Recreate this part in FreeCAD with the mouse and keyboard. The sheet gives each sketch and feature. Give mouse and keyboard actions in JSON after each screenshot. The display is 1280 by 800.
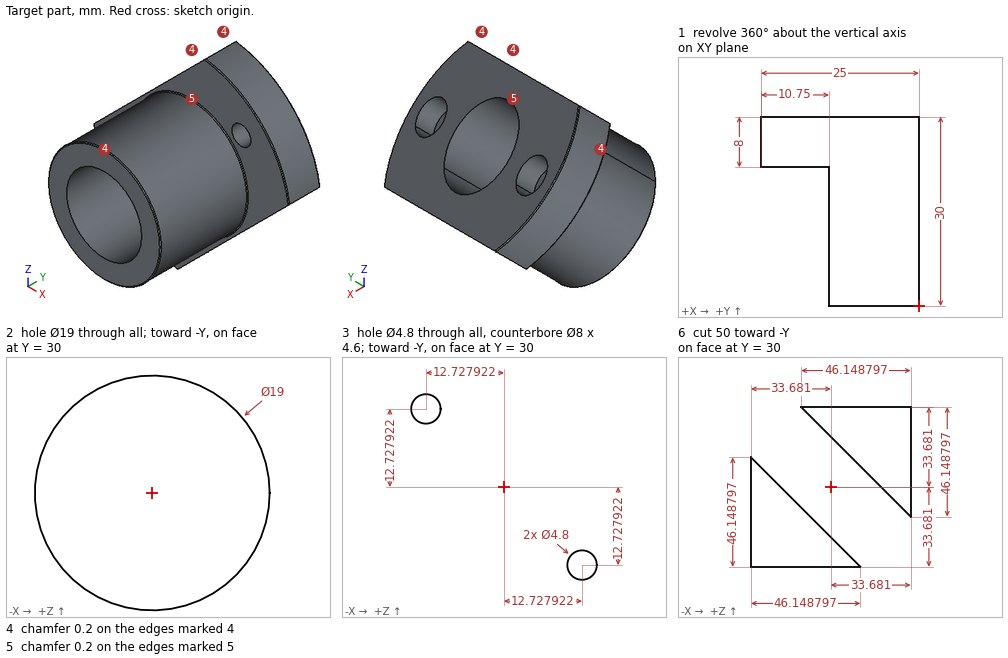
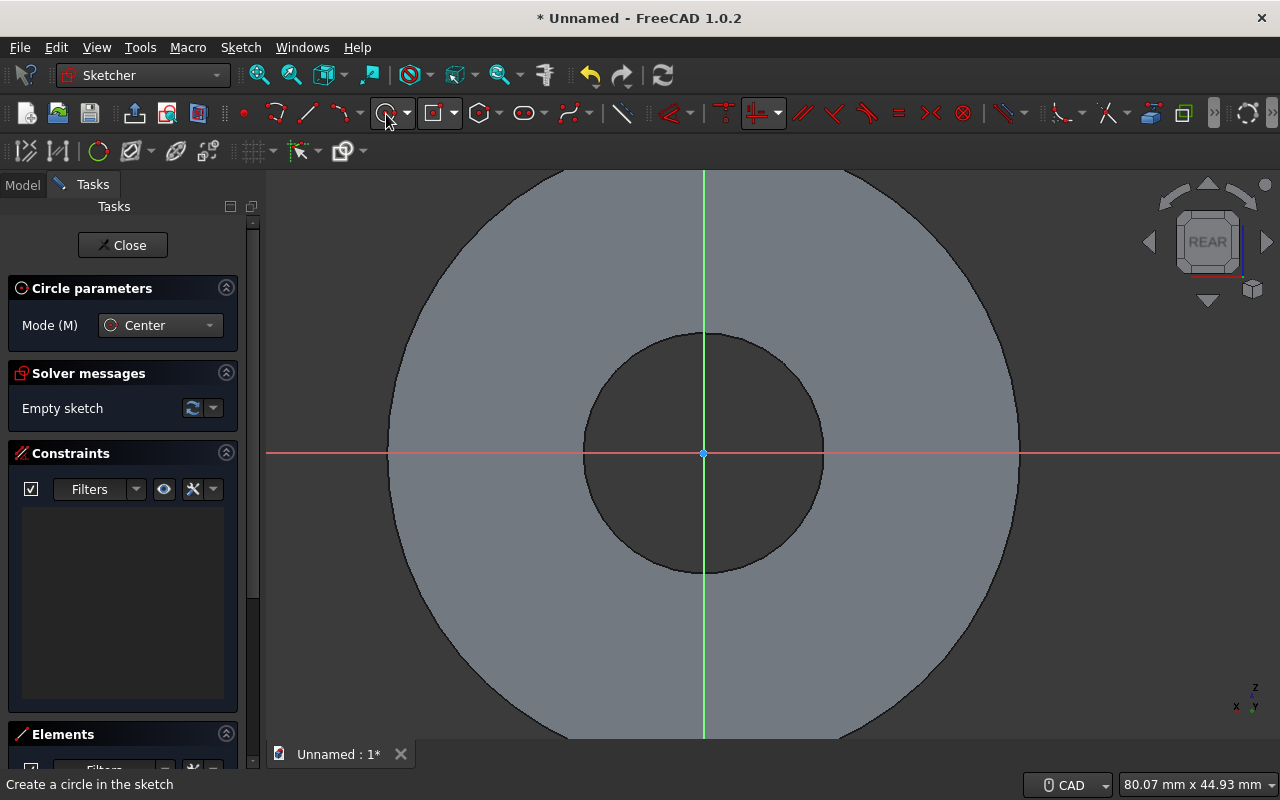
{"action": "left_click", "coordinate": [865, 614]}
{"action": "mouse_move", "coordinate": [886, 593]}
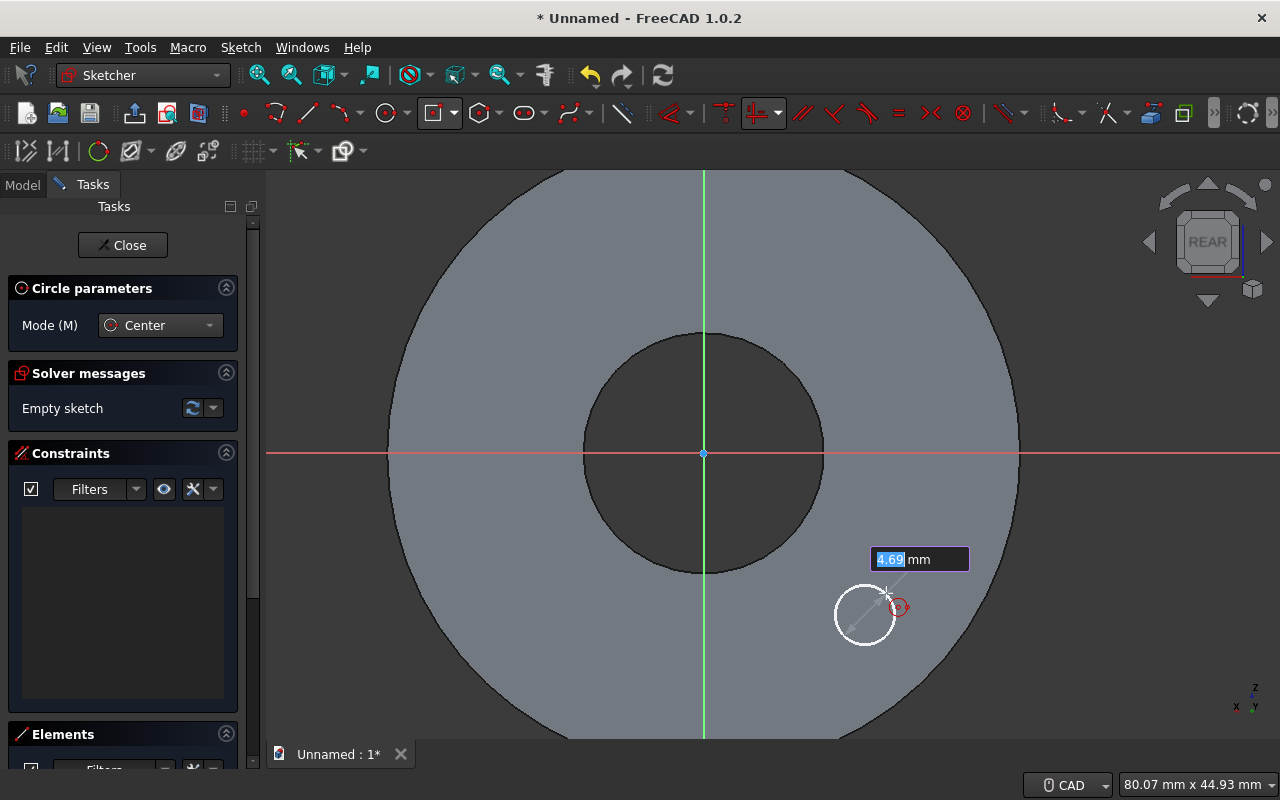
{"action": "type", "text": "4.8"}
{"action": "key", "text": "Return"}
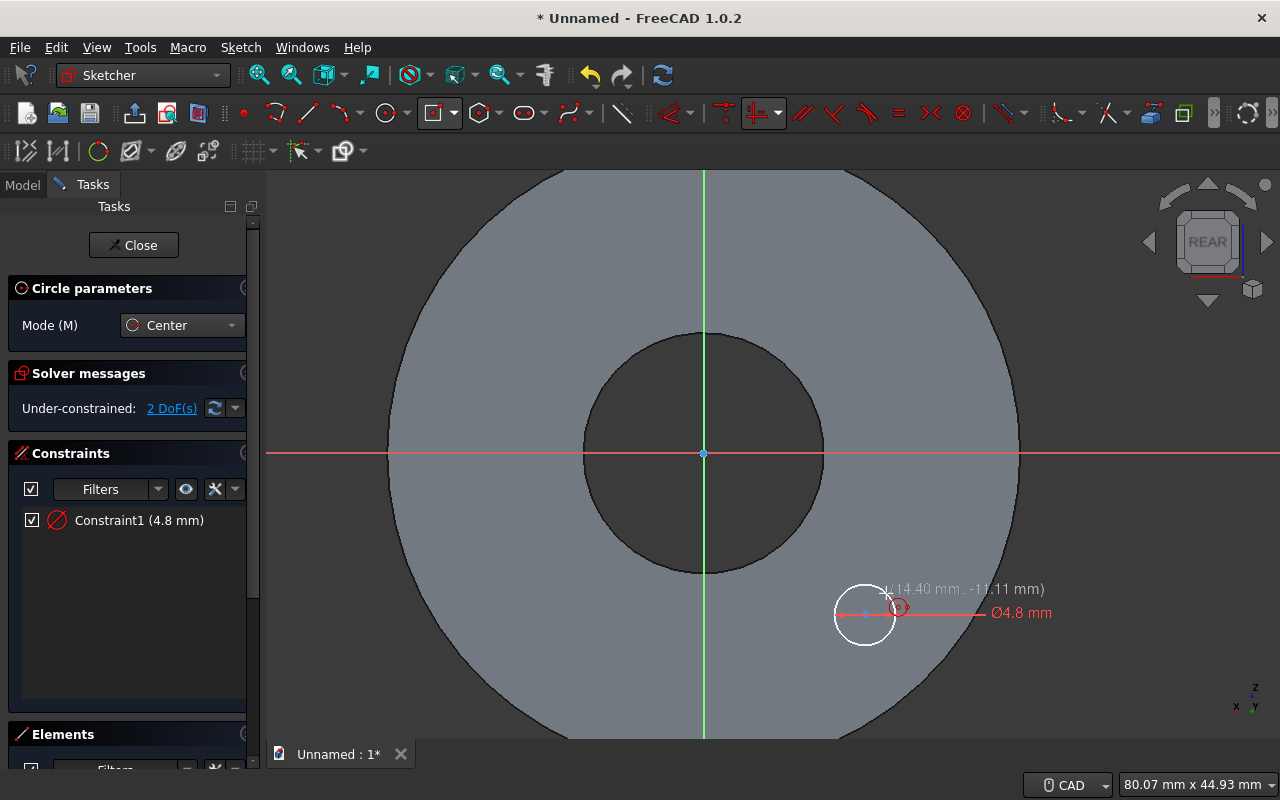
{"action": "left_click", "coordinate": [543, 292]}
{"action": "mouse_move", "coordinate": [564, 271]}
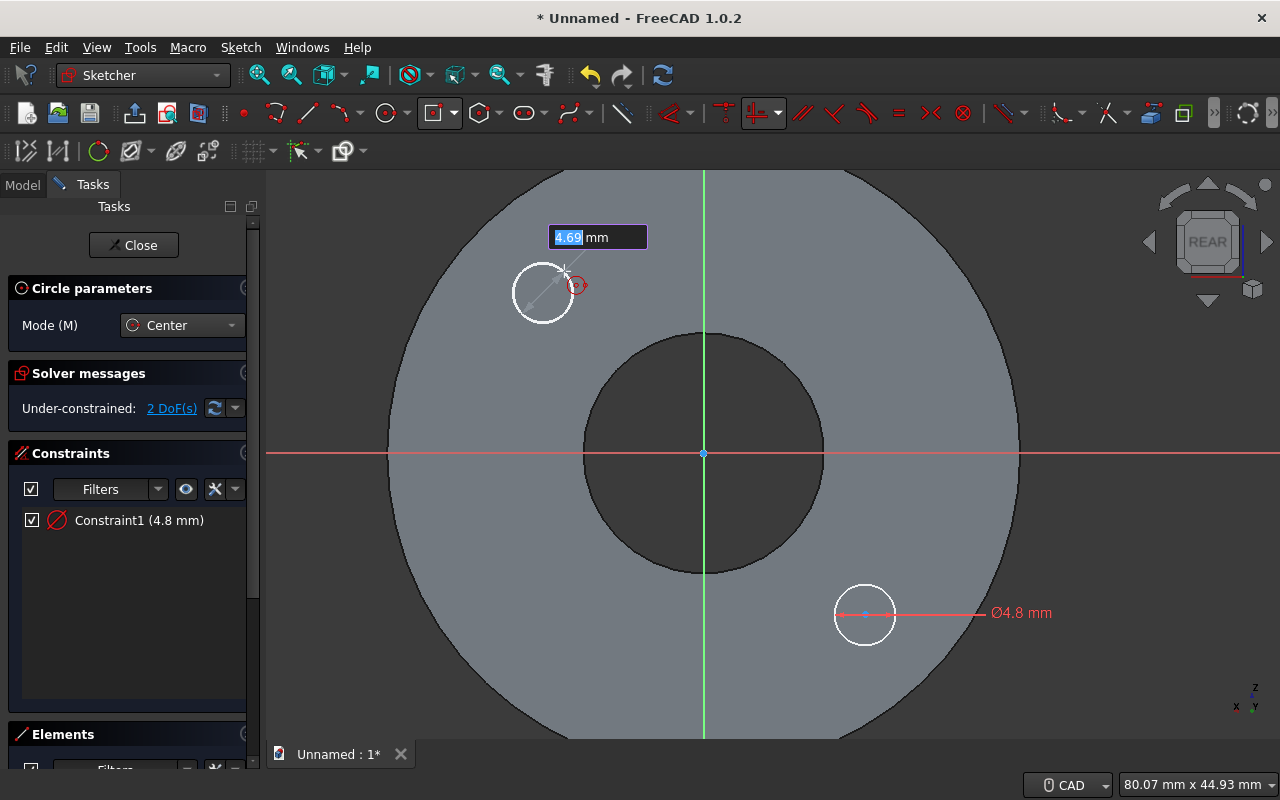
{"action": "type", "text": "4.8"}
{"action": "key", "text": "Return"}
{"action": "key", "text": "Escape"}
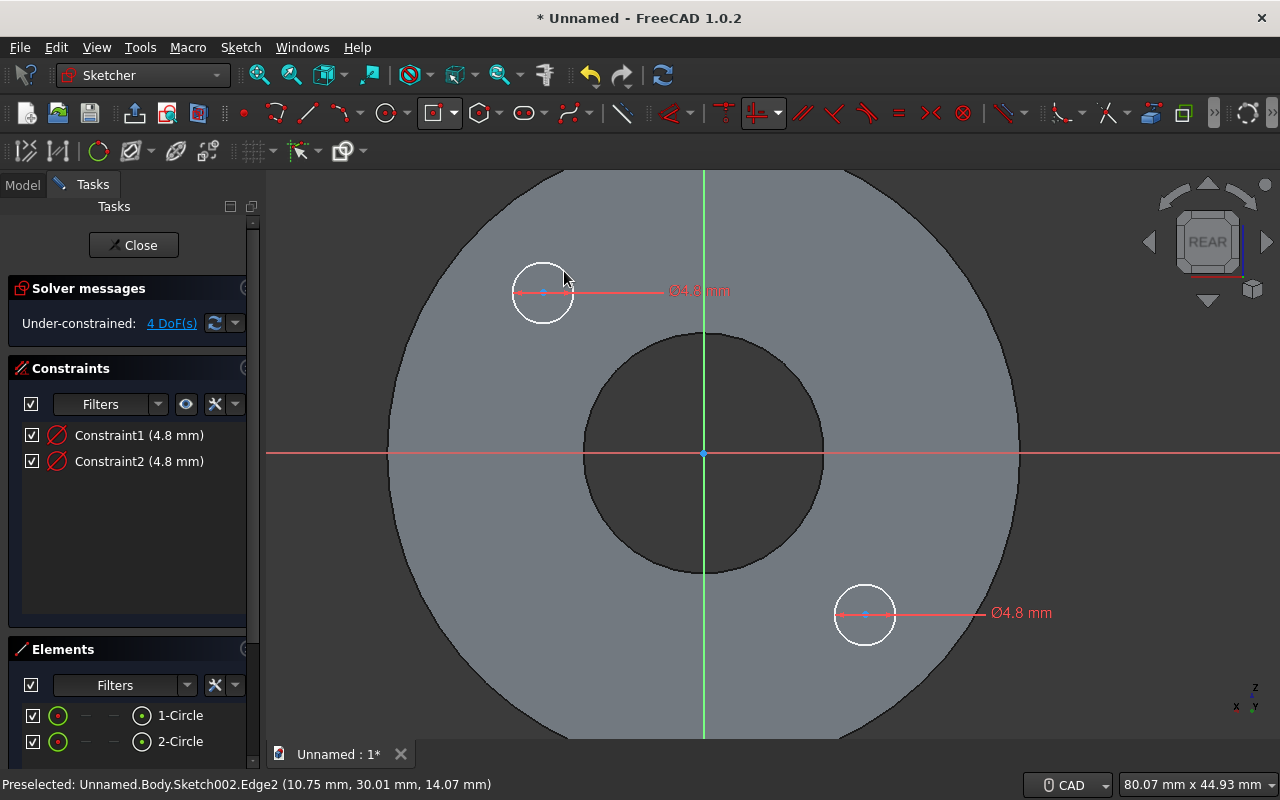
{"action": "left_click", "coordinate": [670, 114]}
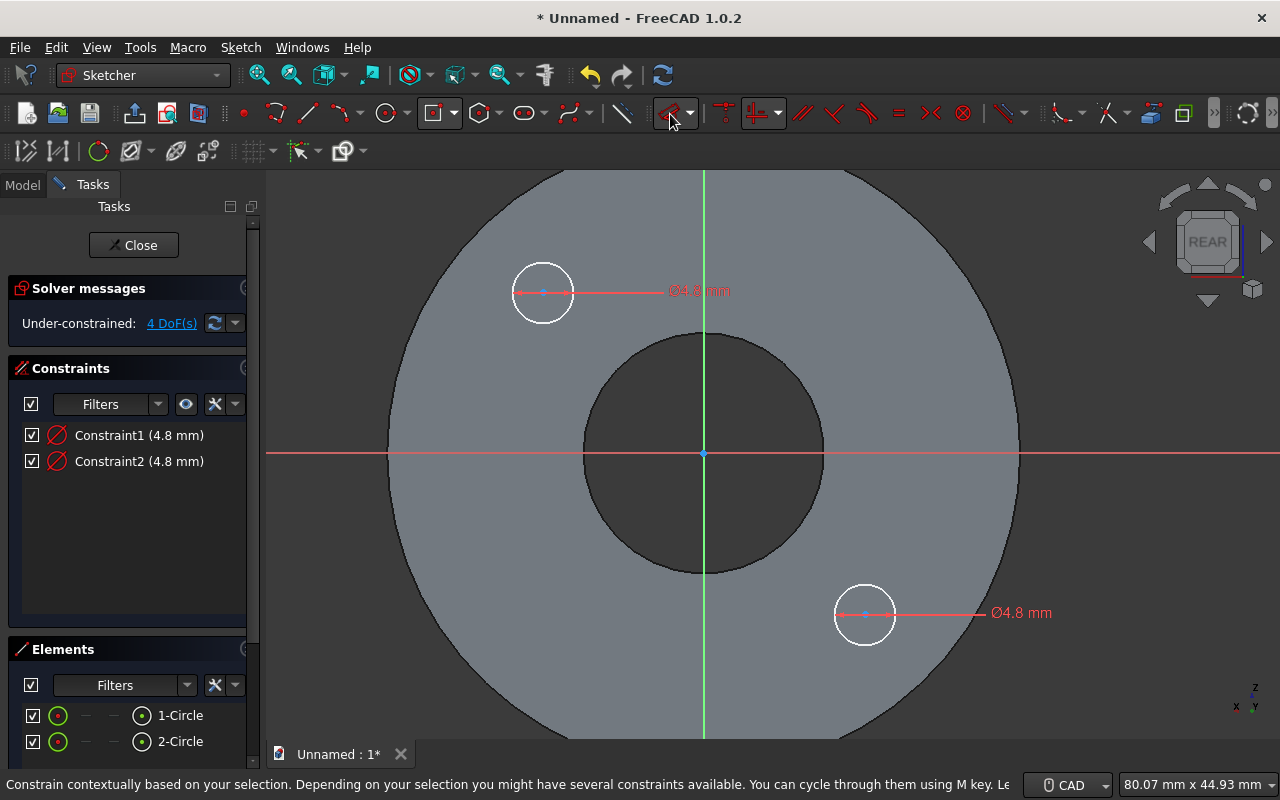
{"action": "left_click", "coordinate": [865, 615]}
{"action": "left_click", "coordinate": [784, 649]}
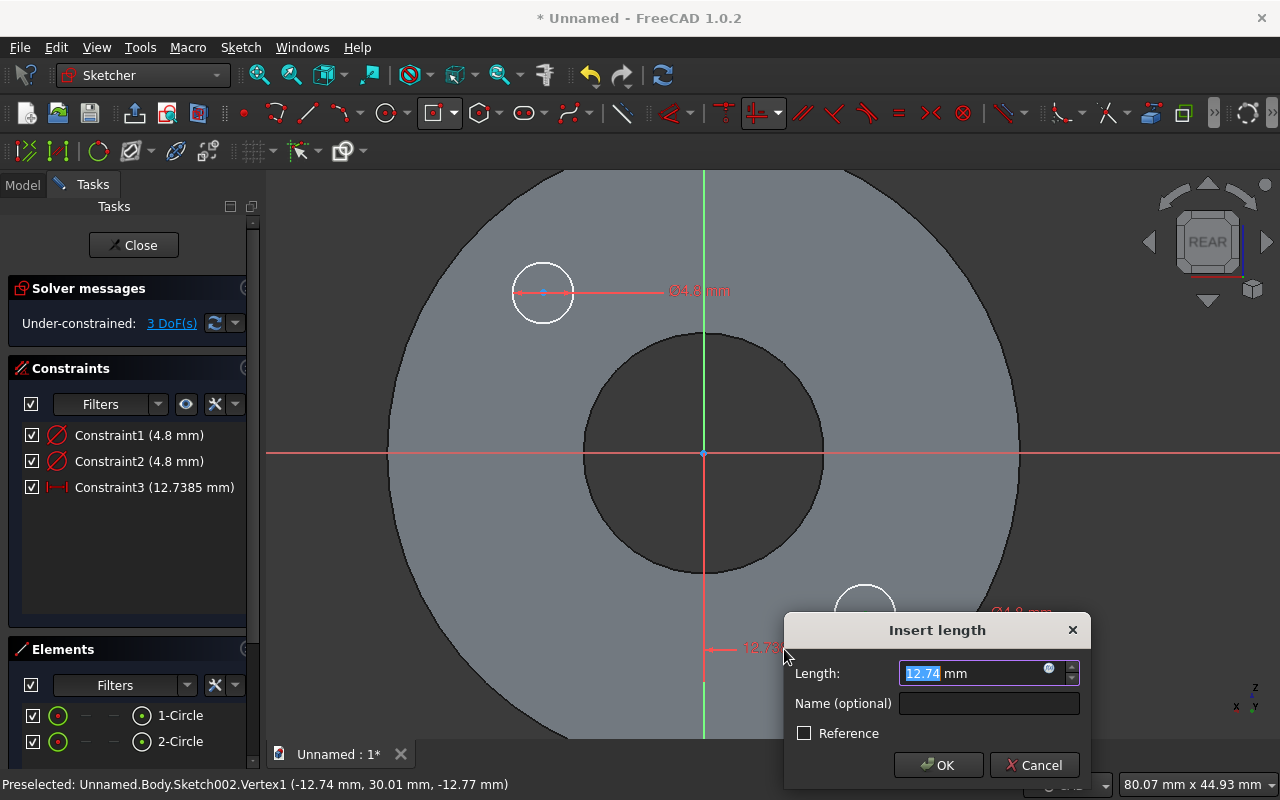
{"action": "type", "text": "12.727922"}
{"action": "key", "text": "Return"}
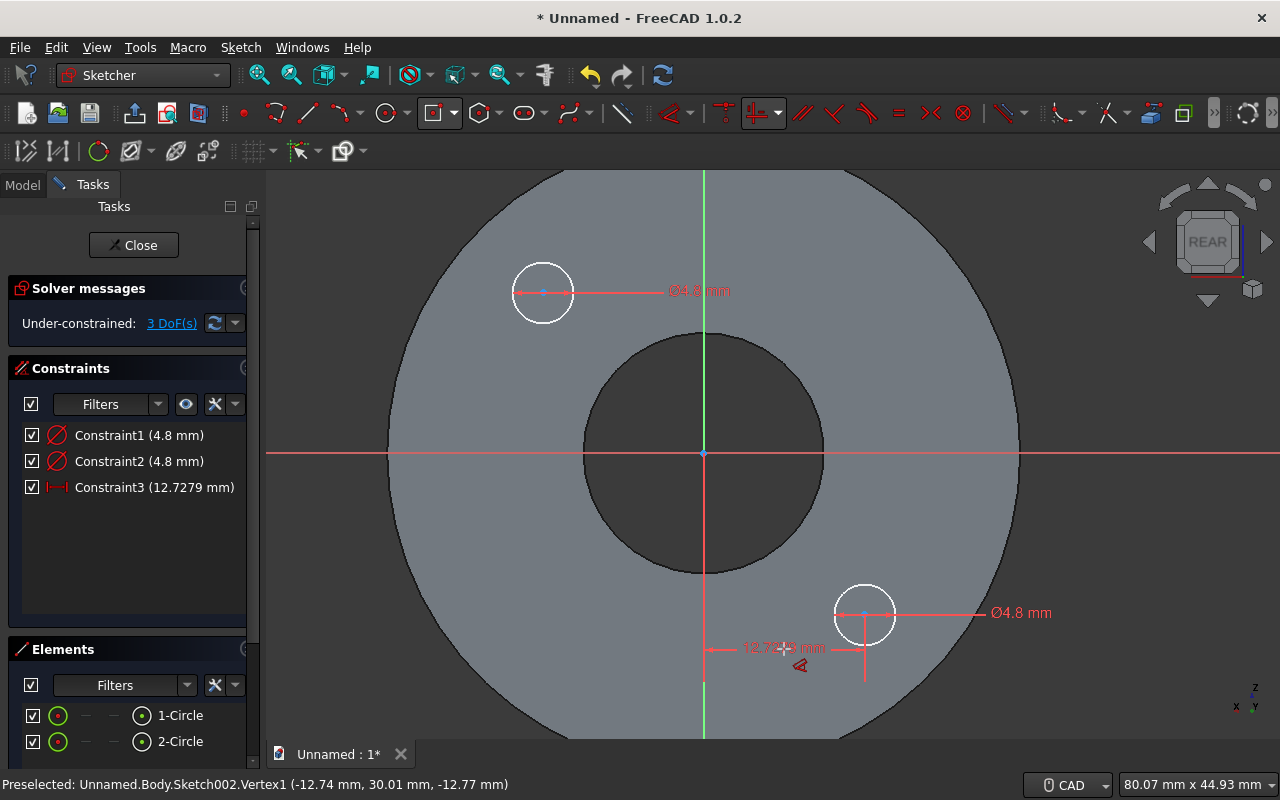
{"action": "left_click", "coordinate": [865, 615]}
{"action": "left_click", "coordinate": [899, 534]}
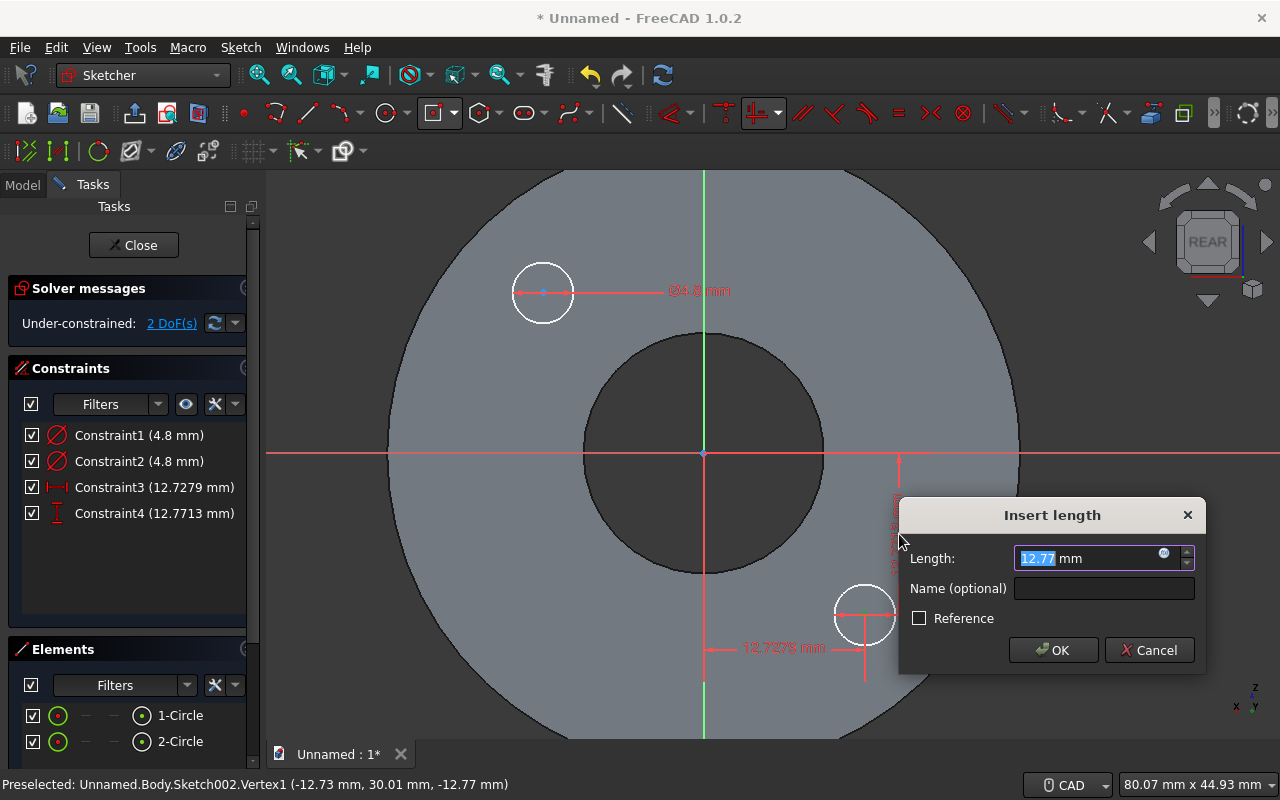
{"action": "type", "text": "12.727922"}
{"action": "key", "text": "Return"}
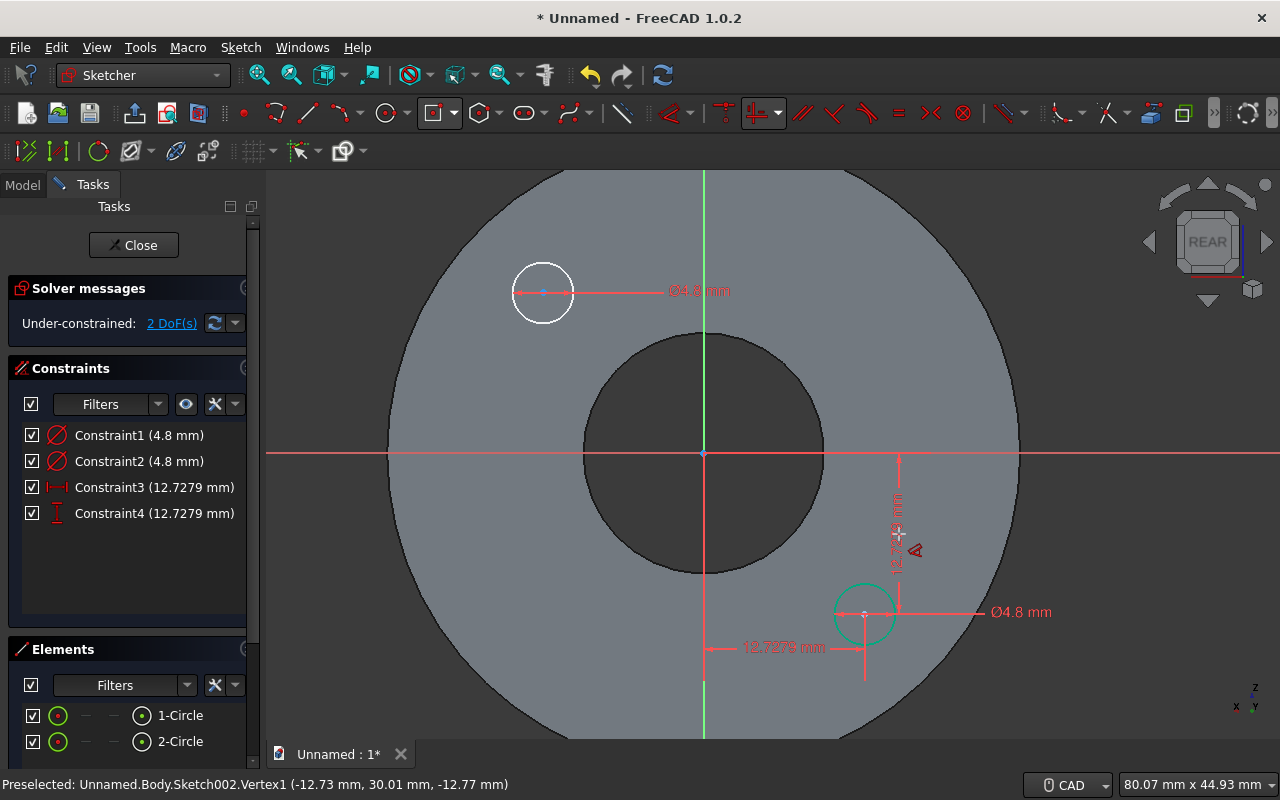
{"action": "left_click", "coordinate": [543, 293]}
{"action": "left_click", "coordinate": [623, 259]}